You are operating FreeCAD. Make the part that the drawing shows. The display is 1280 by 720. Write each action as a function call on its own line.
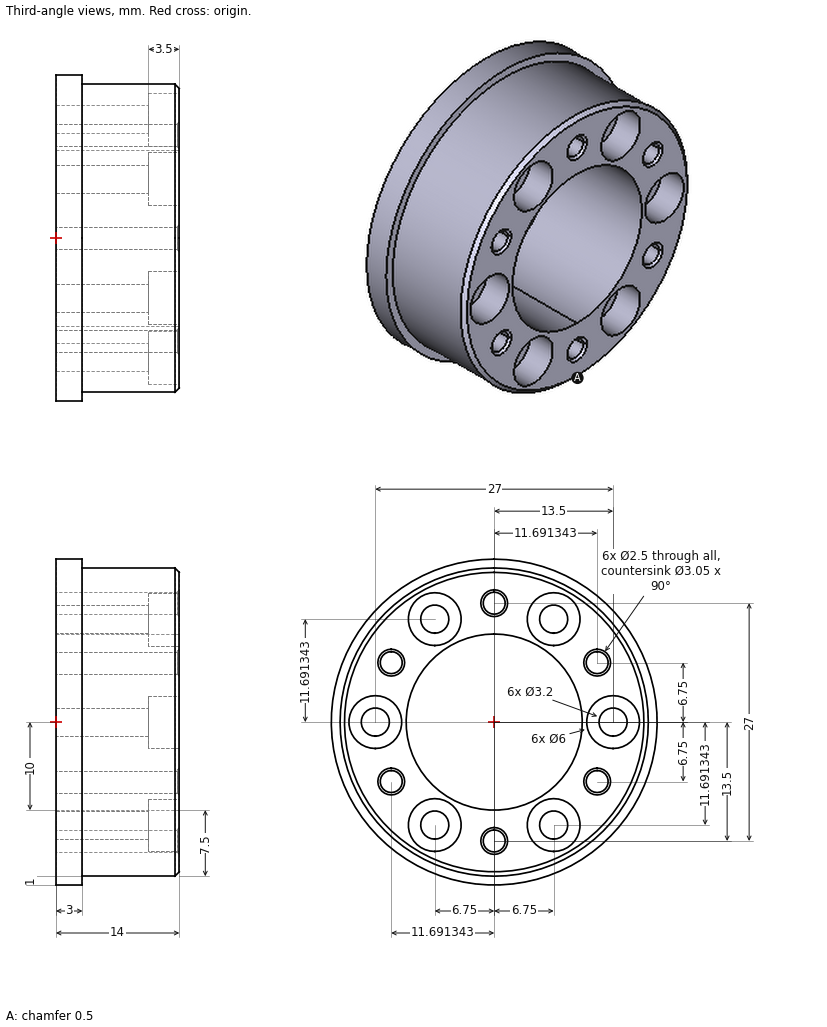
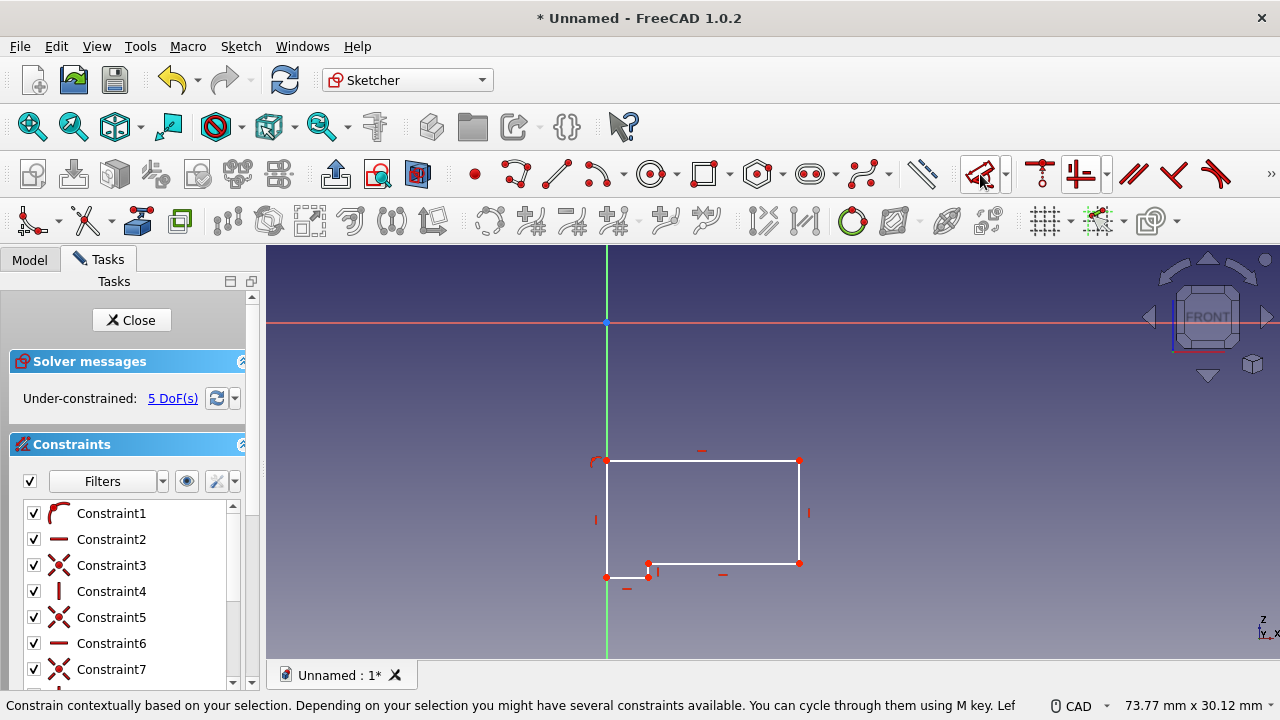
scroll(648, 571, up, 6)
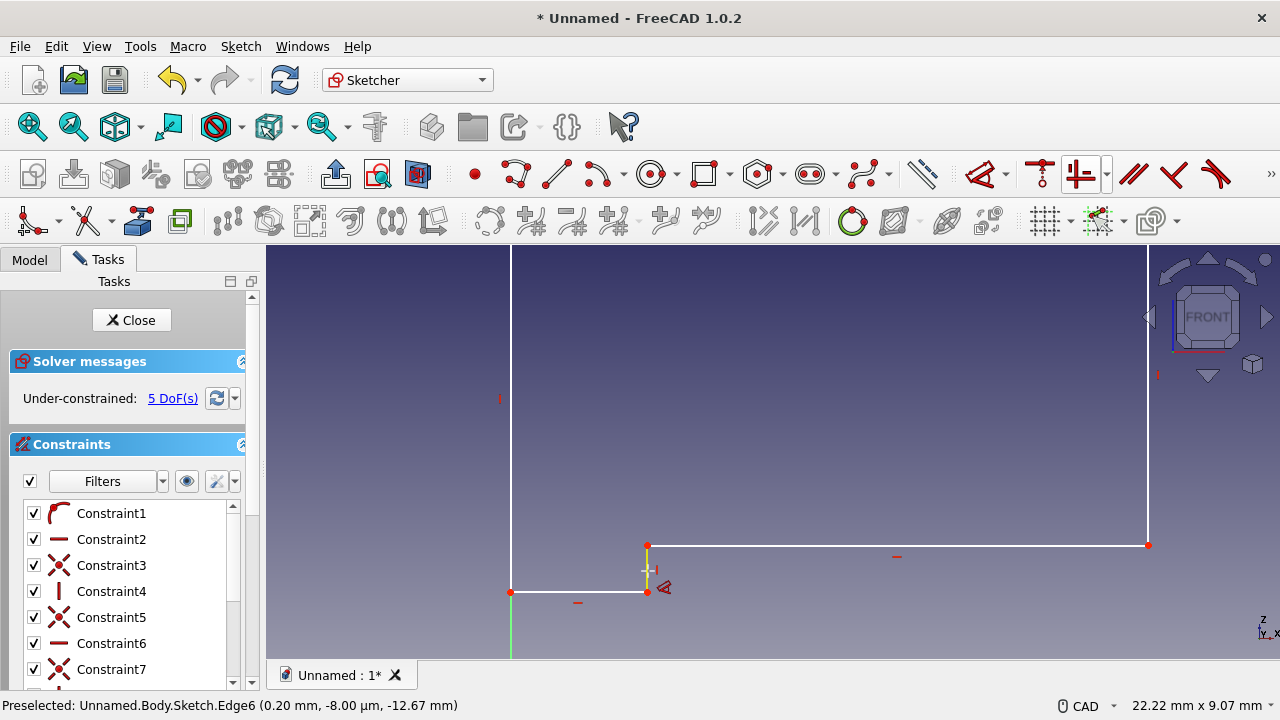
click(647, 569)
click(613, 569)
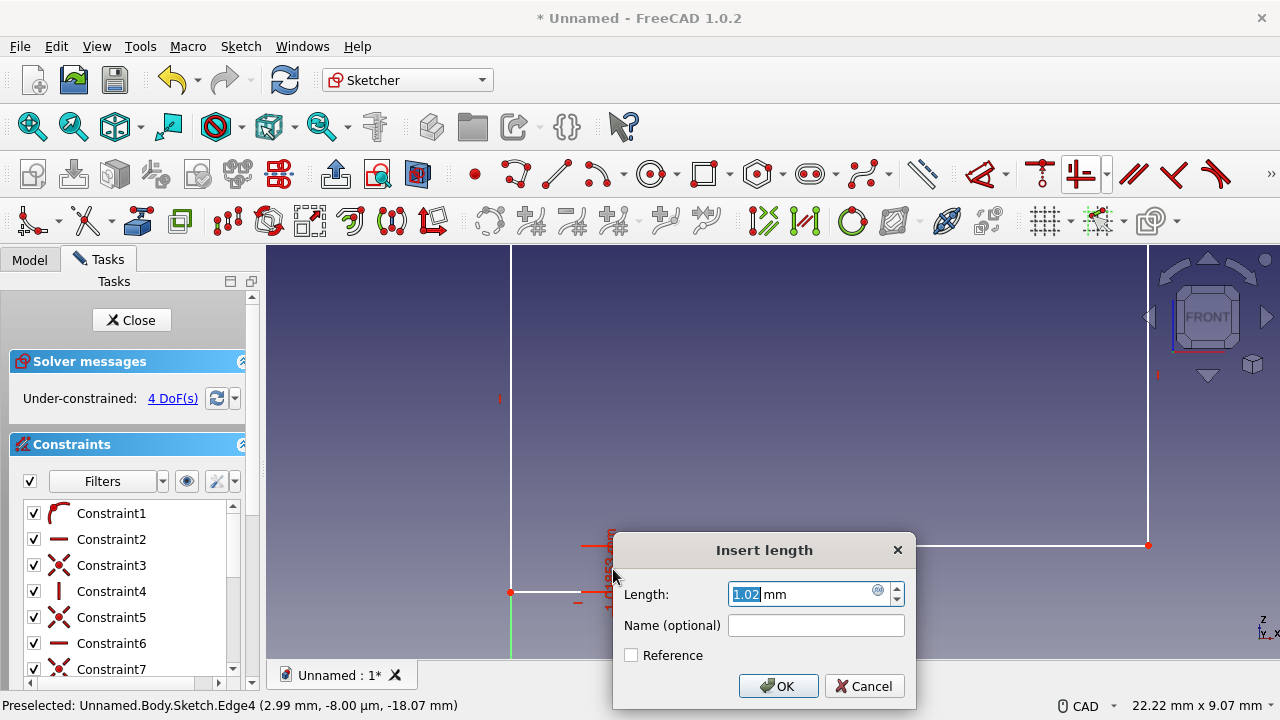
text(1)
key(Return)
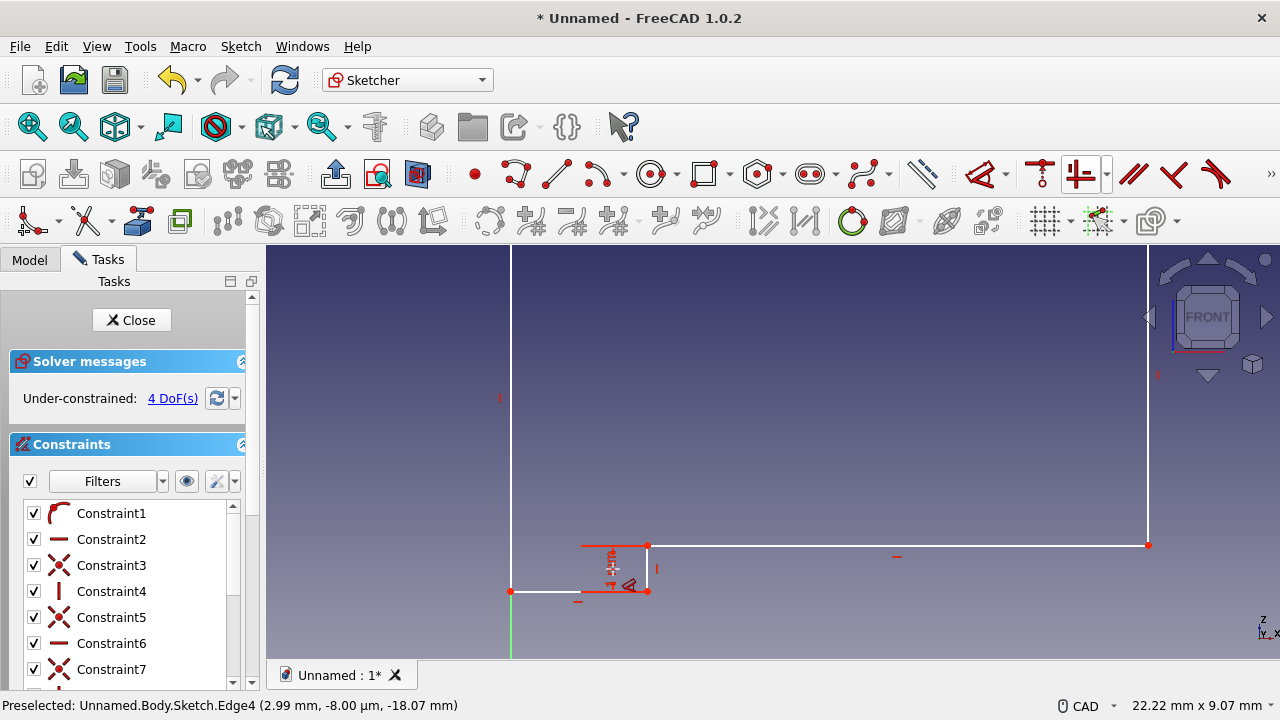
click(606, 592)
click(579, 626)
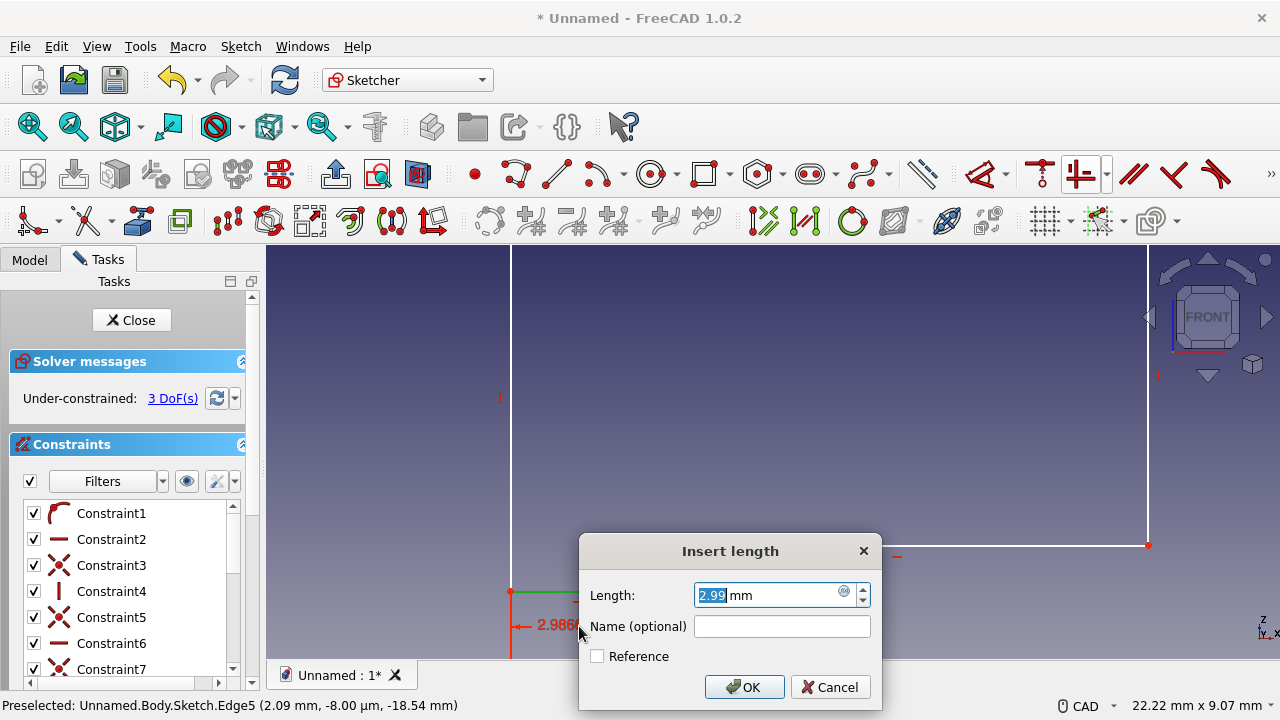
text(3)
key(Return)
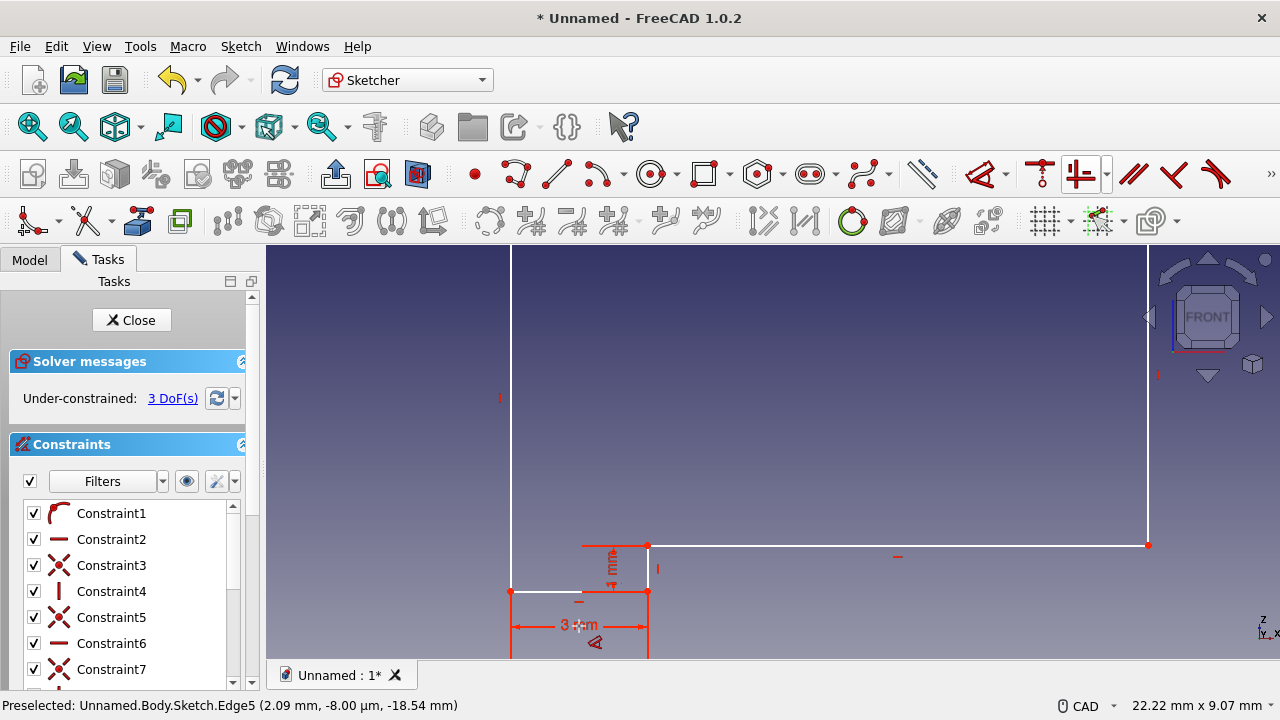
scroll(650, 575, down, 6)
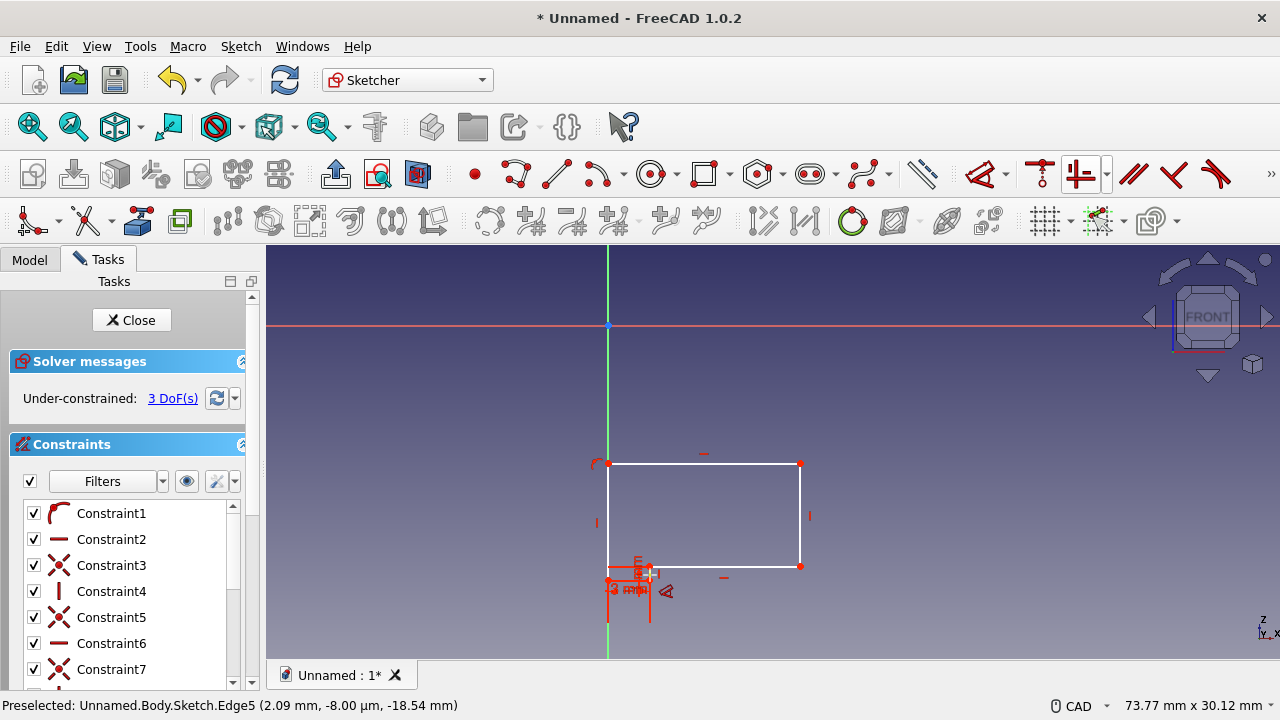
click(666, 464)
click(704, 498)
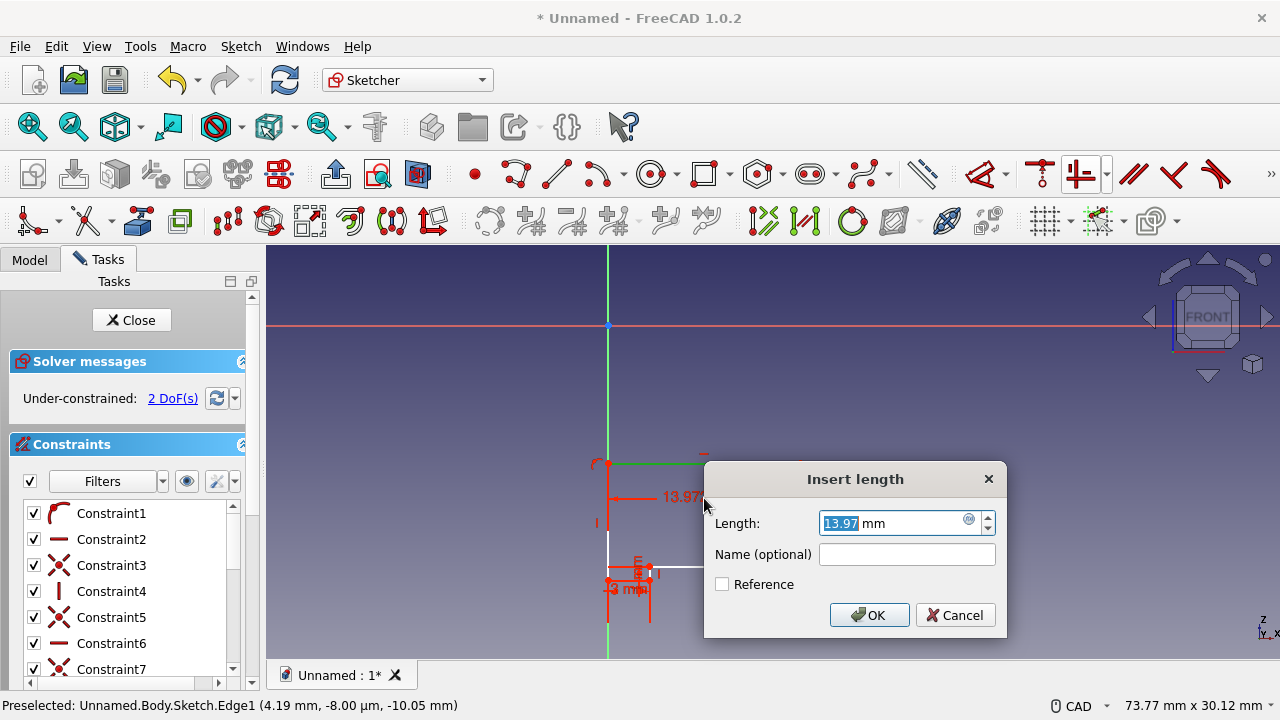
text(14)
key(Return)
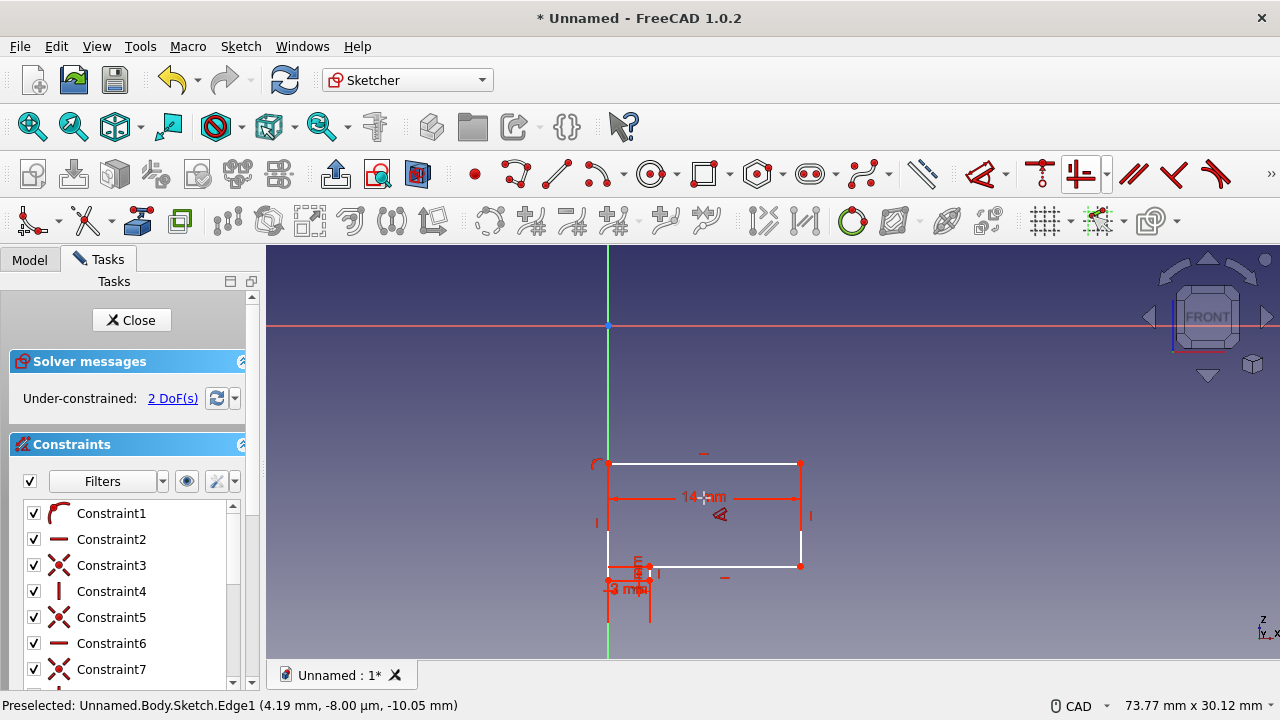
click(801, 495)
click(835, 515)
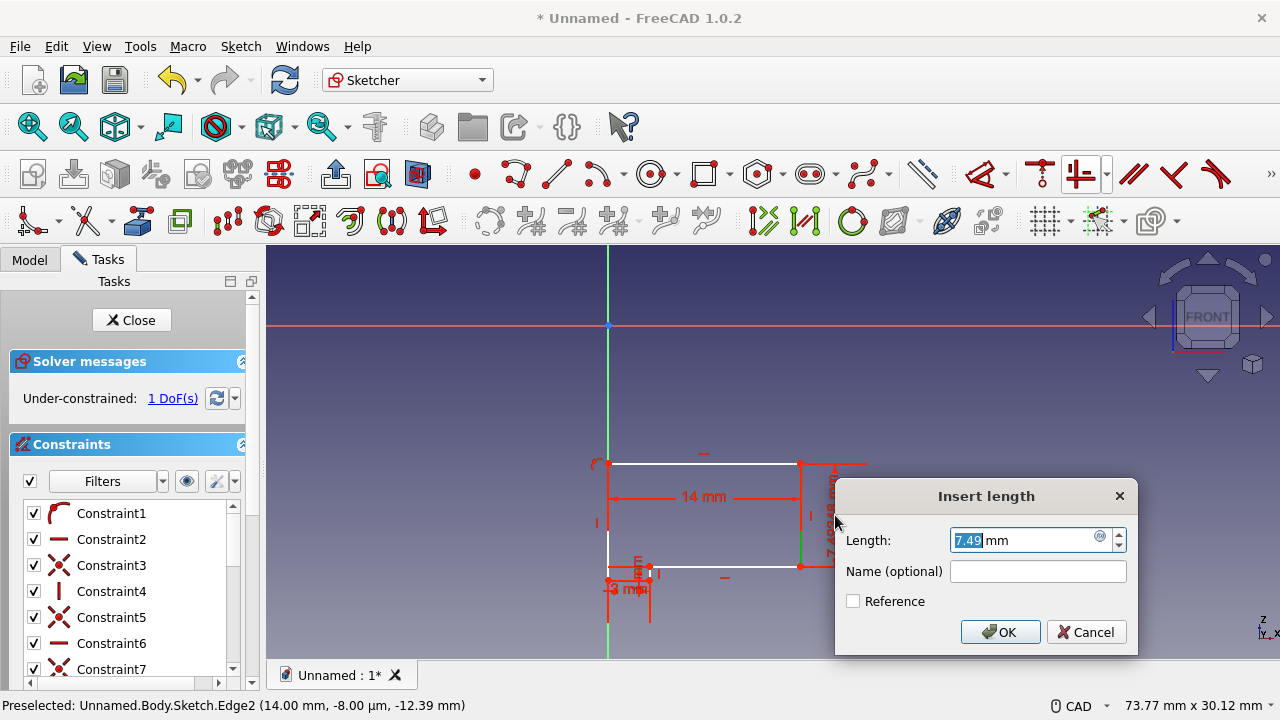
text(7.5)
key(Return)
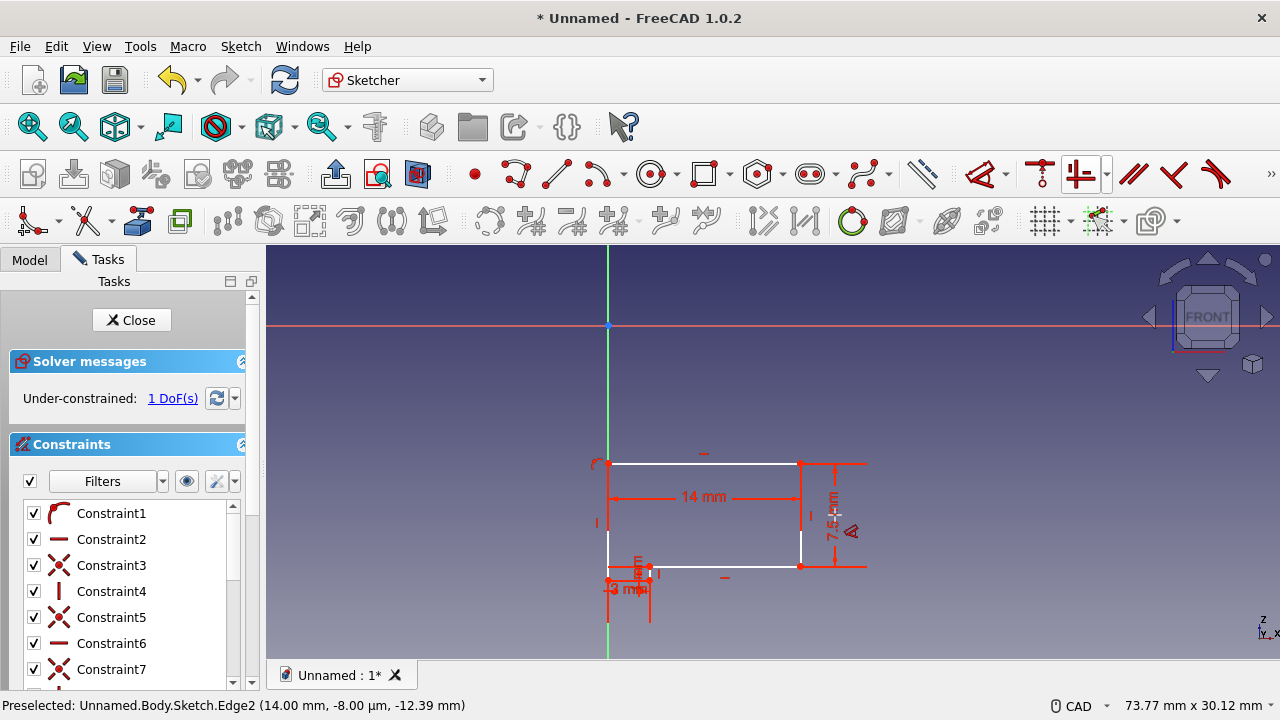
click(608, 464)
click(574, 395)